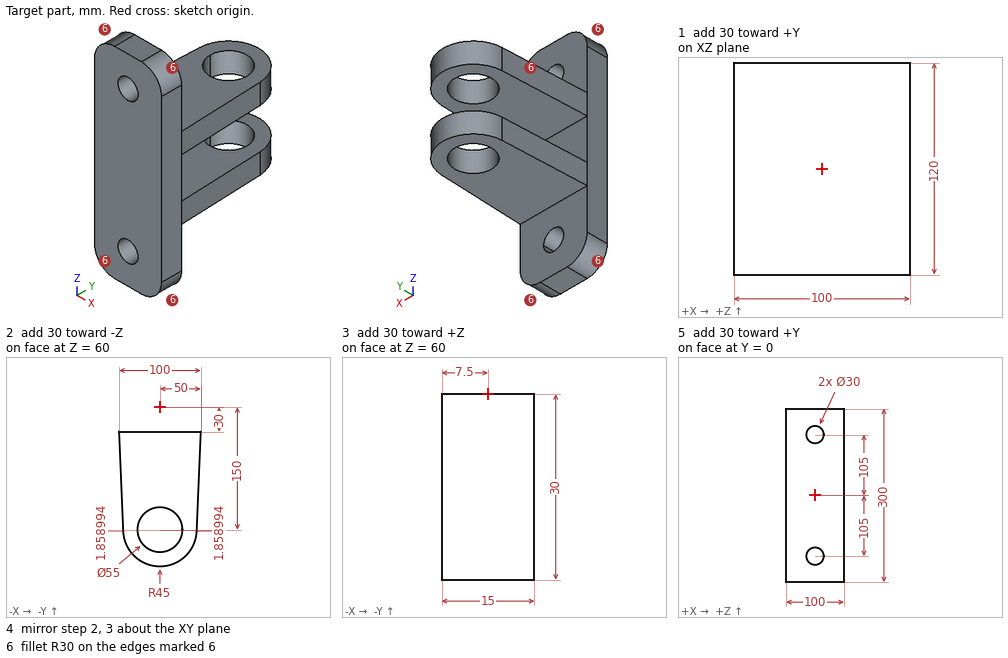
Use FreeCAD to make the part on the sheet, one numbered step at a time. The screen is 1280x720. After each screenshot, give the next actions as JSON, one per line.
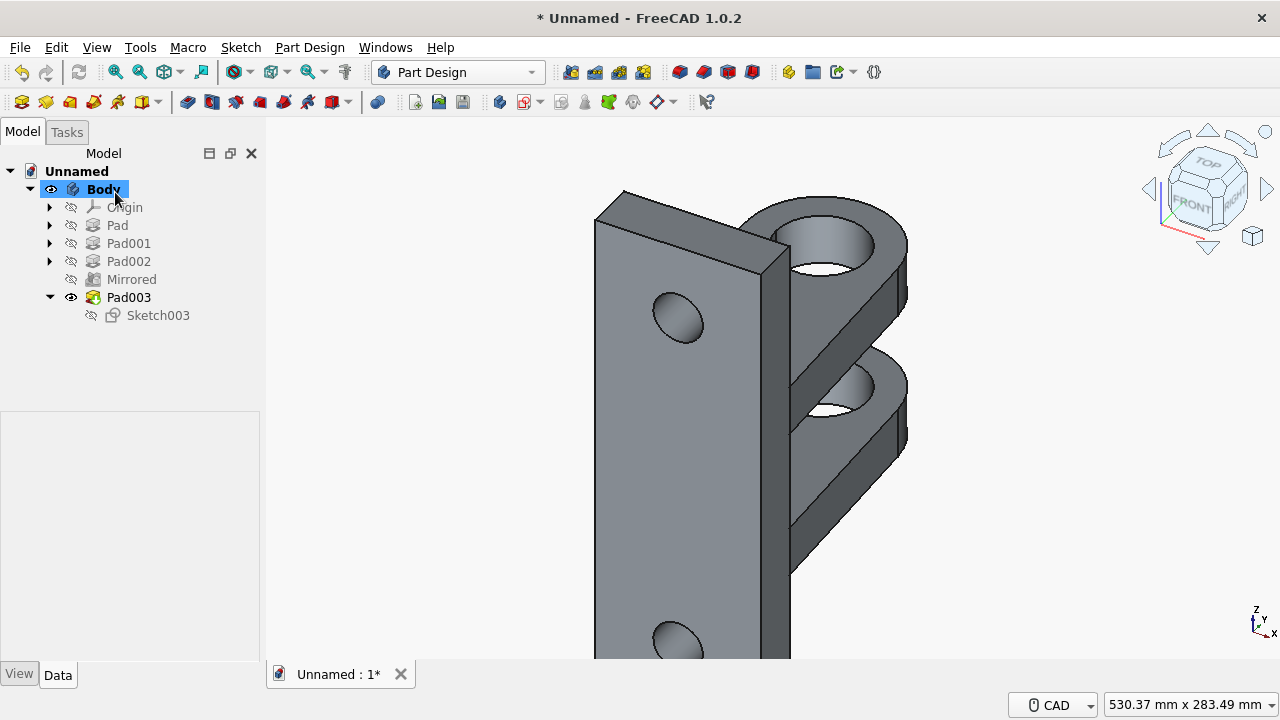
{"action": "left_click", "coordinate": [116, 72]}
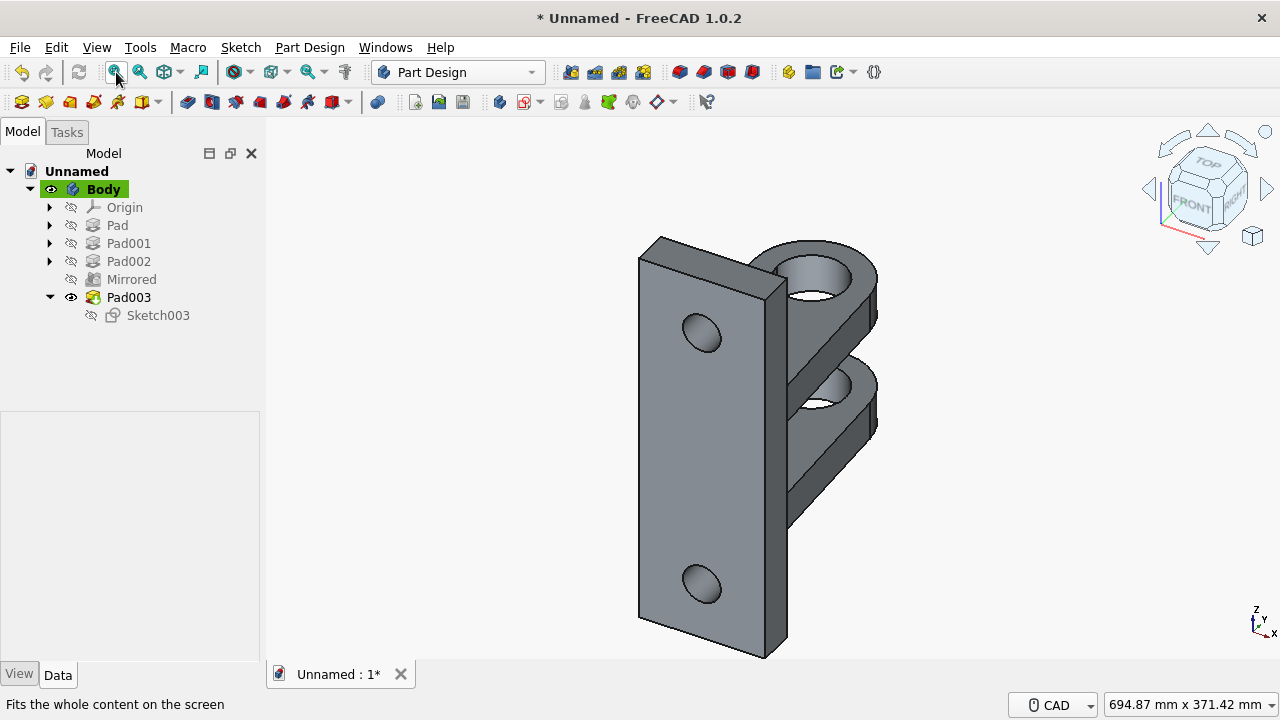
{"action": "left_click", "coordinate": [776, 288]}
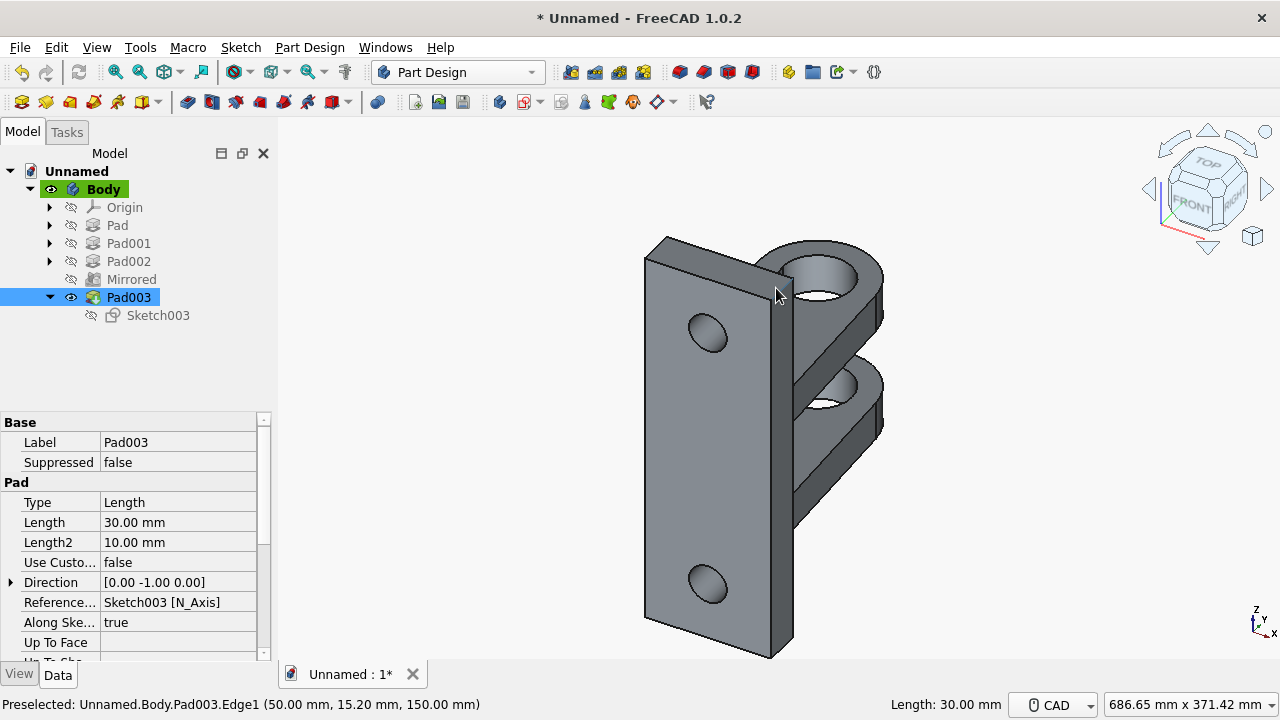
{"action": "key", "text": "0"}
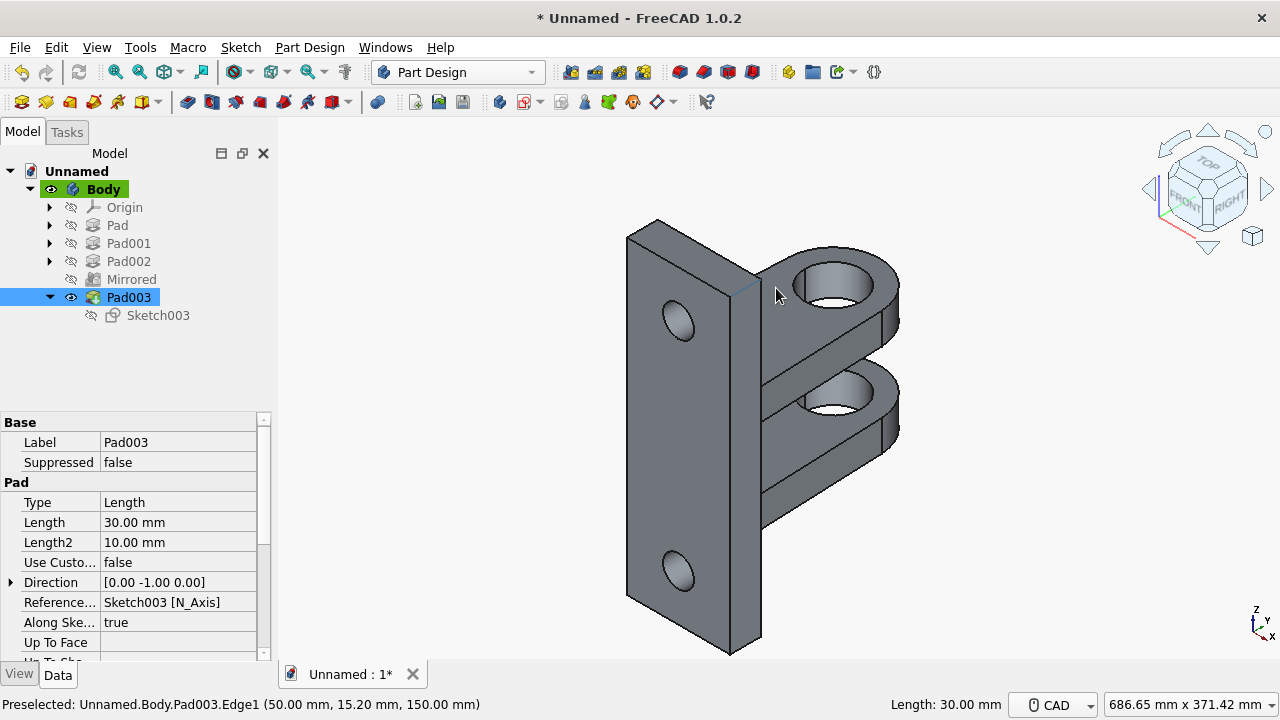
{"action": "key", "text": "2"}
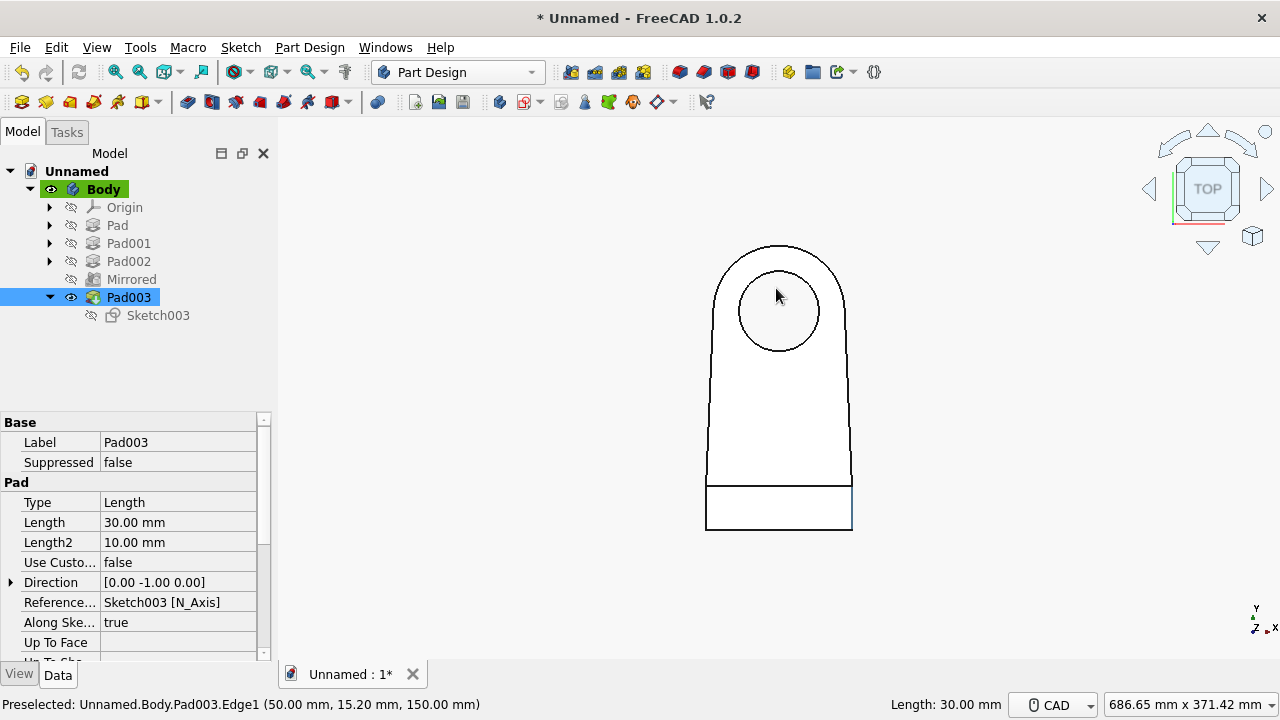
{"action": "left_click", "coordinate": [706, 507], "text": "ctrl"}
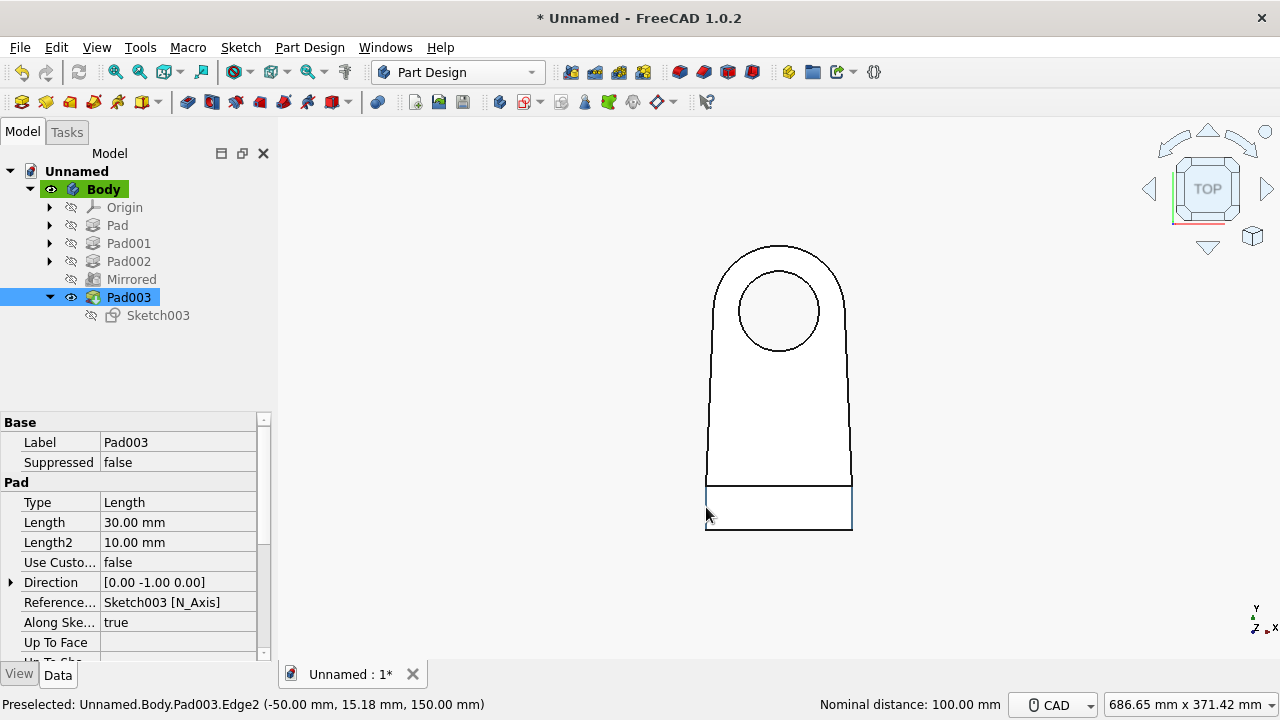
{"action": "key", "text": "1"}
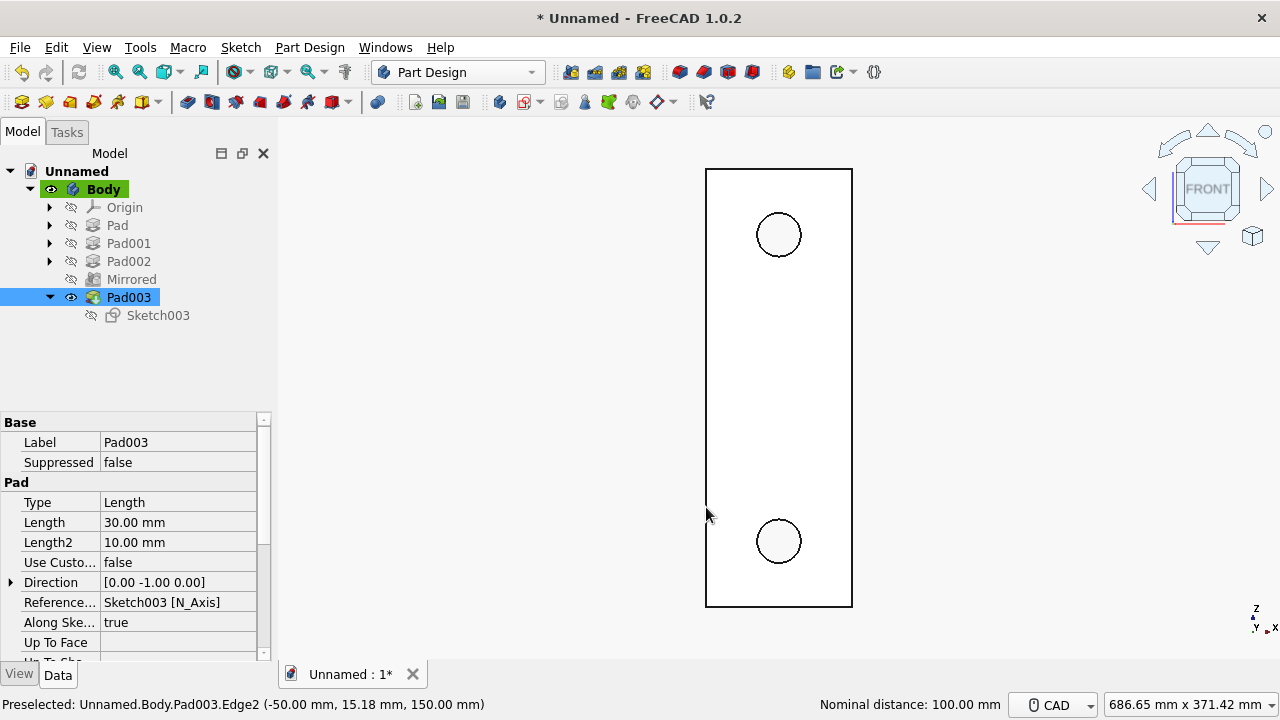
{"action": "key", "text": "3"}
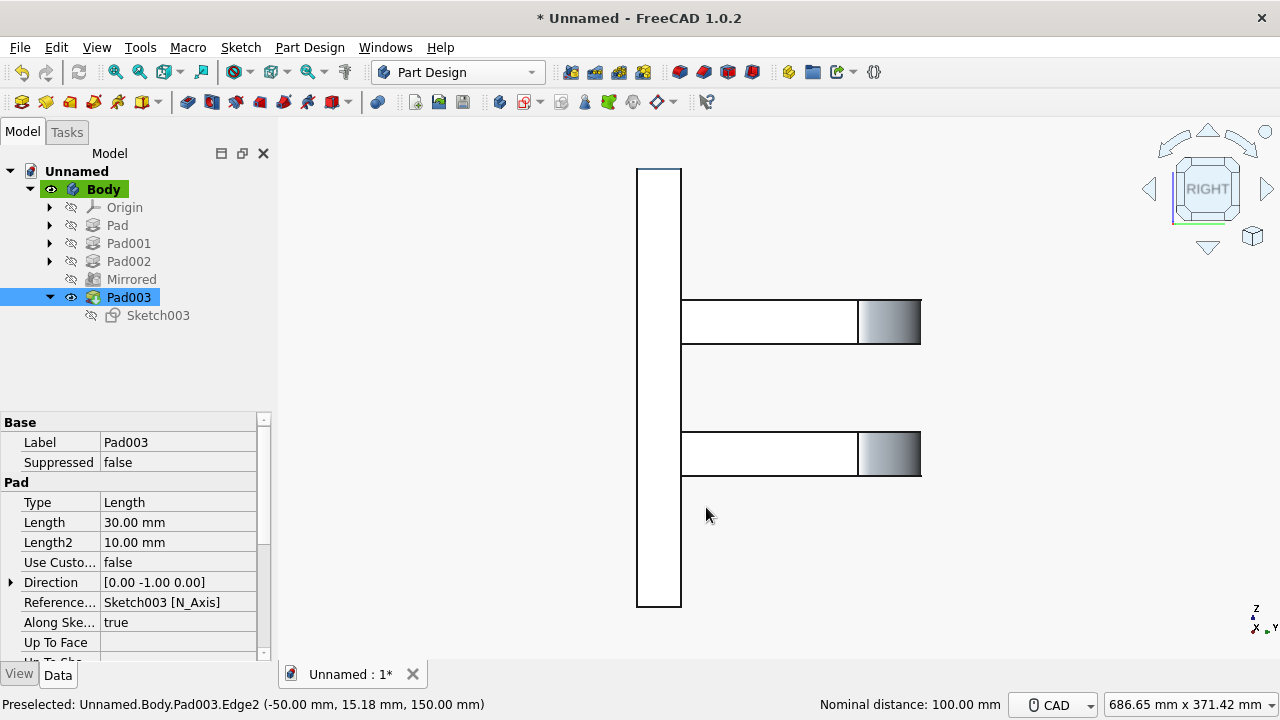
{"action": "left_click", "coordinate": [659, 606], "text": "ctrl"}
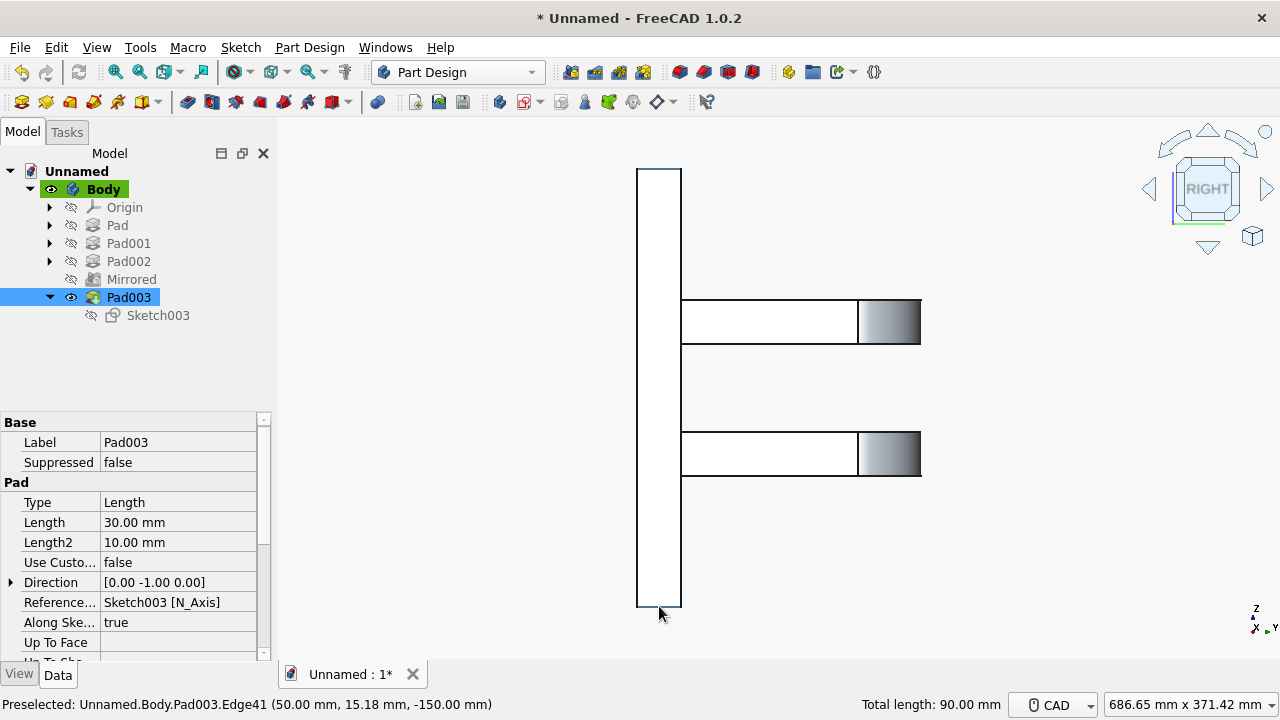
{"action": "key", "text": "5"}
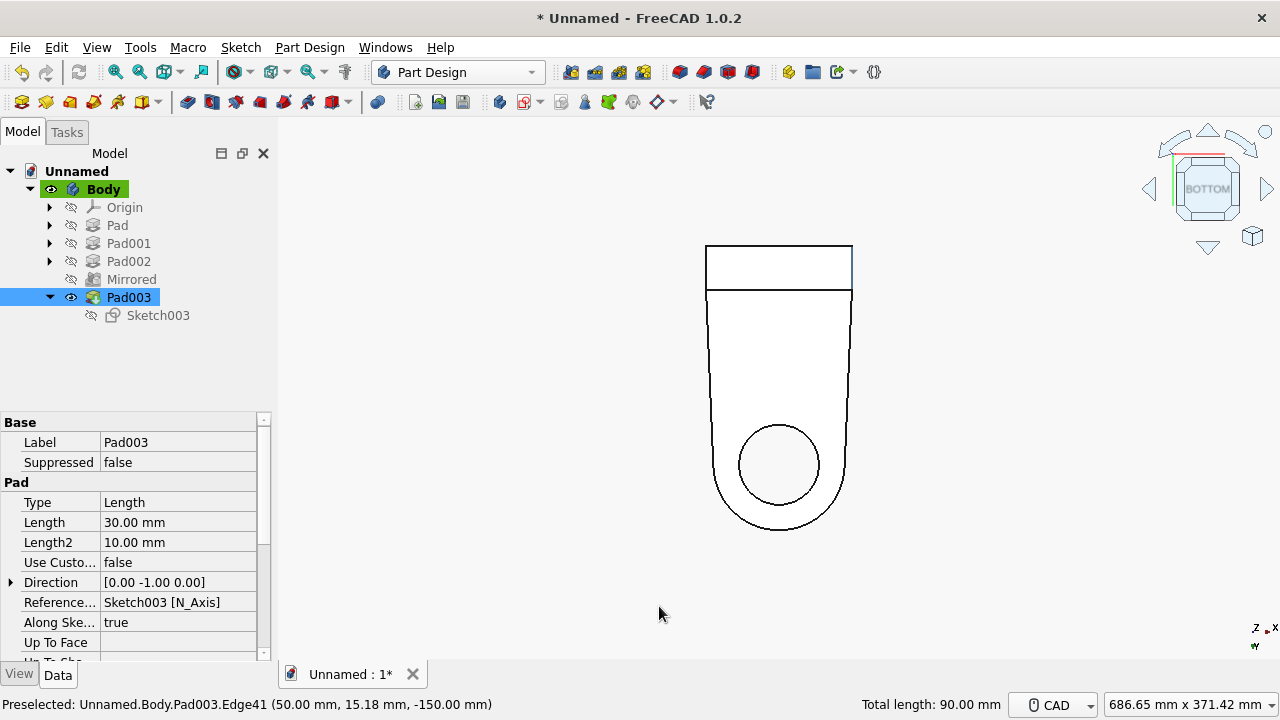
{"action": "left_click", "coordinate": [706, 267], "text": "ctrl"}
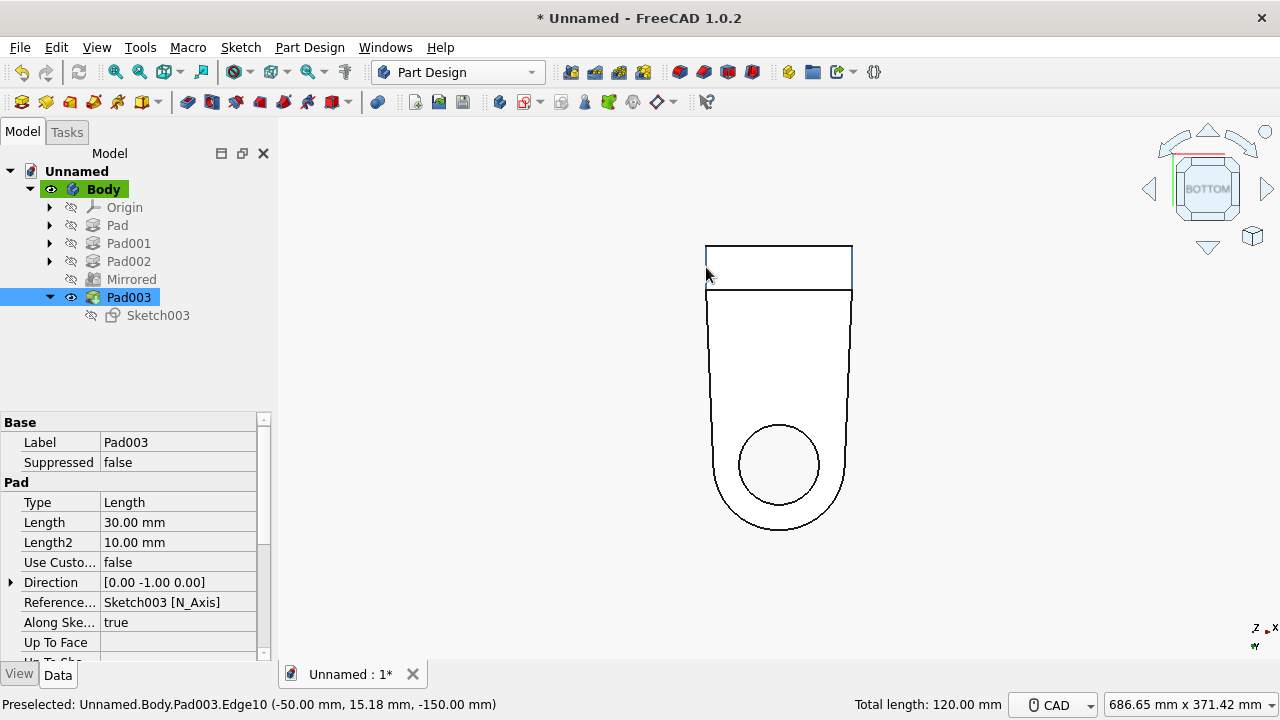
{"action": "left_click", "coordinate": [680, 72]}